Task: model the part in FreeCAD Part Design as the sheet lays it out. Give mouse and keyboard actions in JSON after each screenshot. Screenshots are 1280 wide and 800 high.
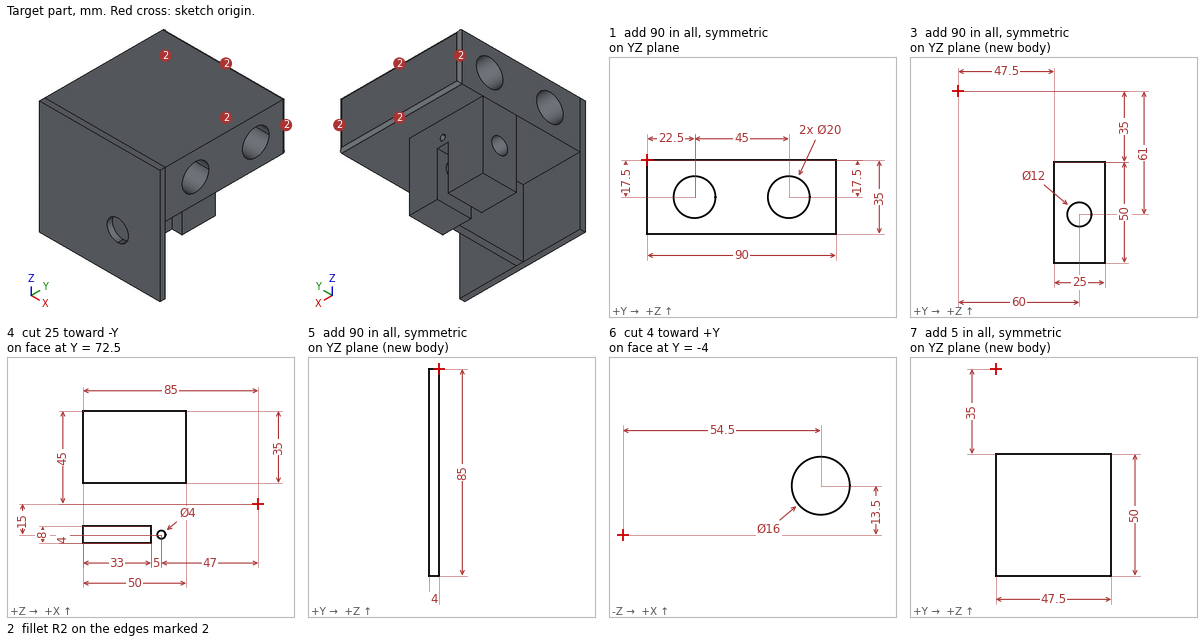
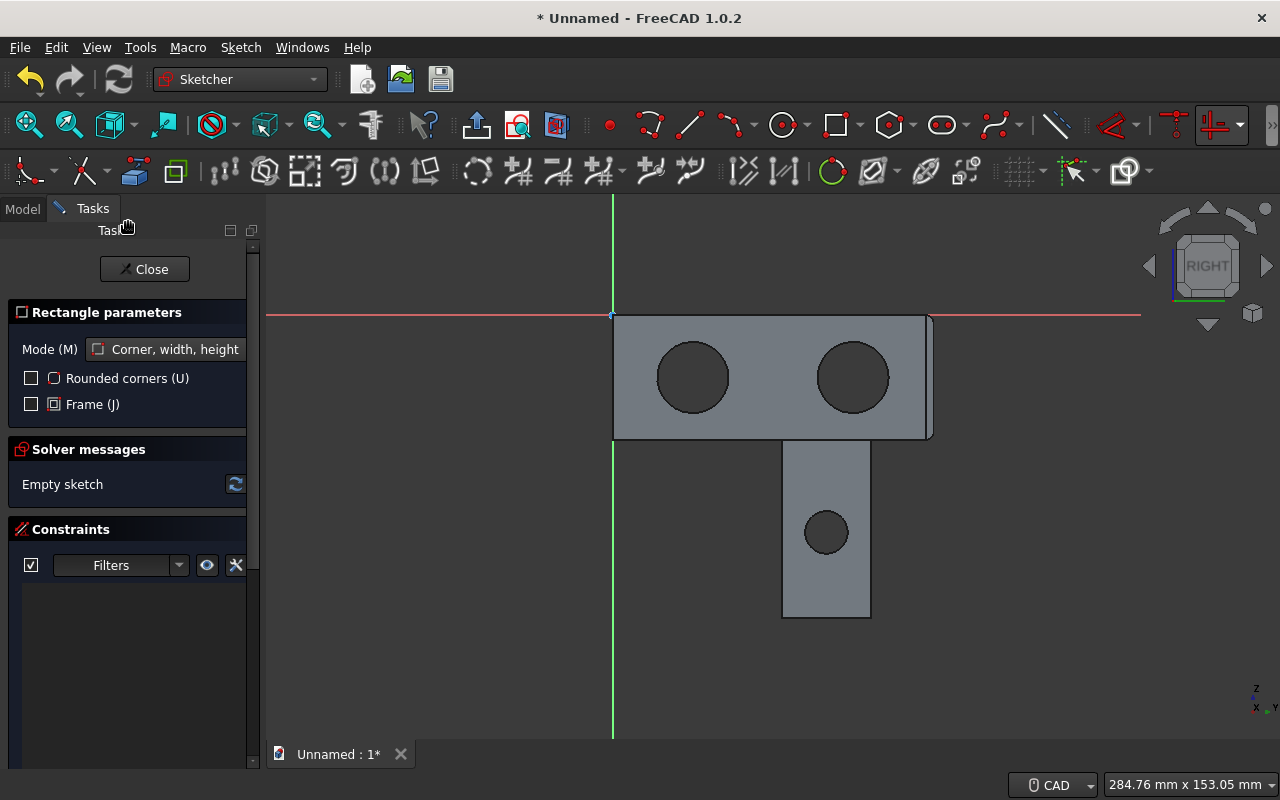
{"action": "left_click", "coordinate": [613, 315]}
{"action": "mouse_move", "coordinate": [599, 618]}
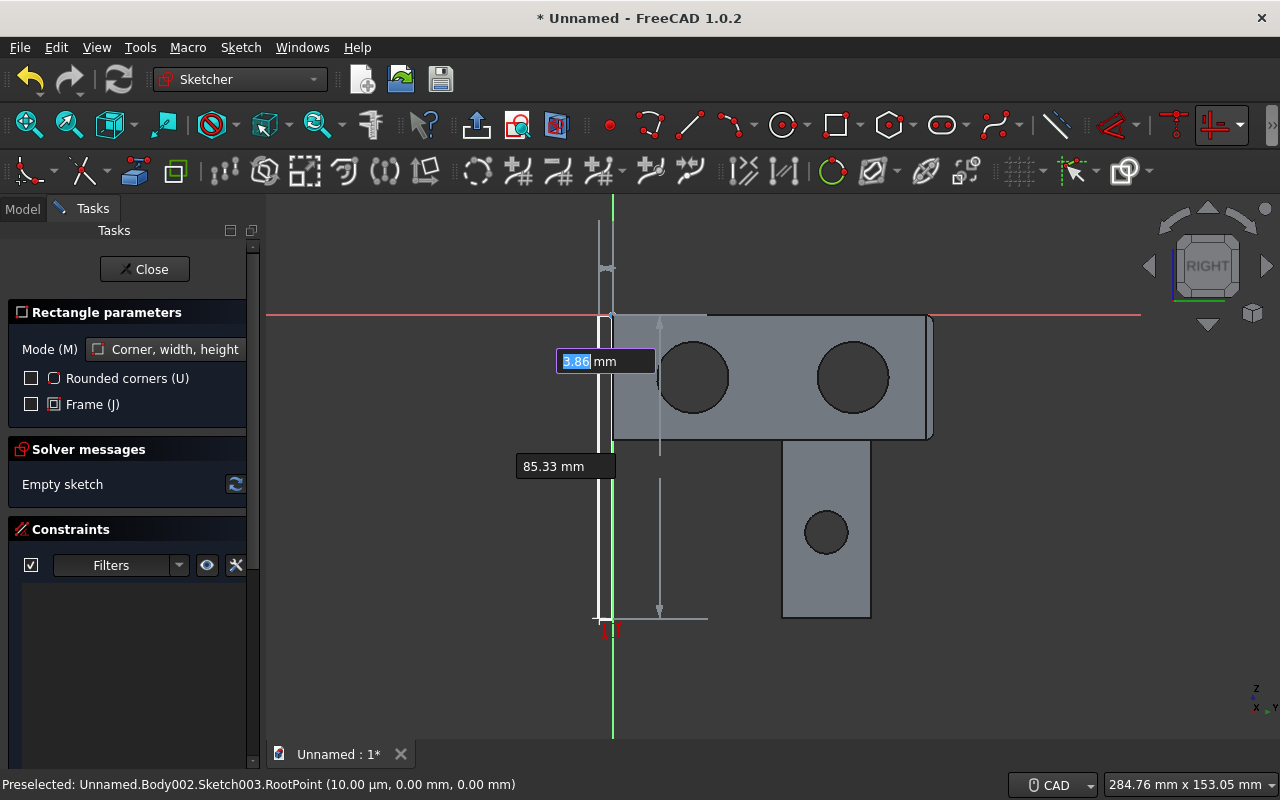
{"action": "type", "text": "4"}
{"action": "key", "text": "Tab"}
{"action": "type", "text": "85"}
{"action": "key", "text": "Return"}
{"action": "key", "text": "Escape"}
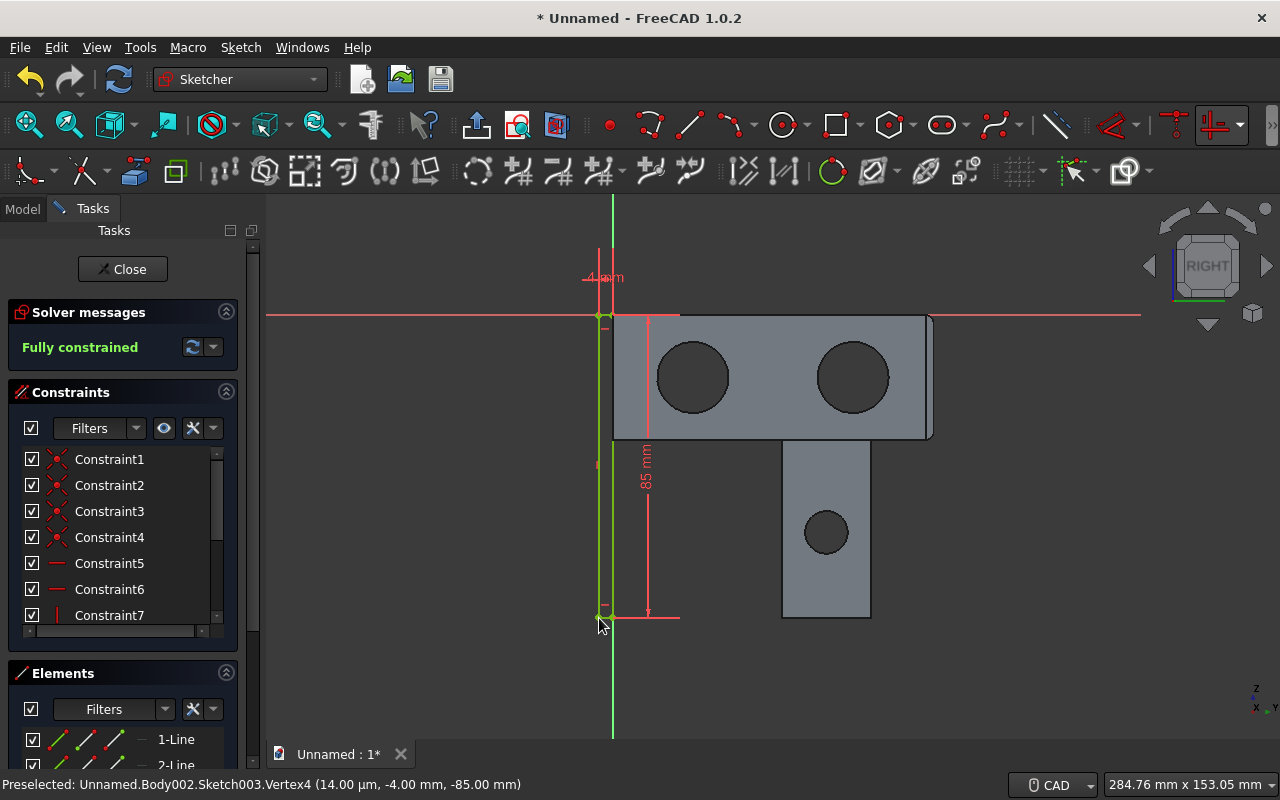
{"action": "left_click", "coordinate": [123, 269]}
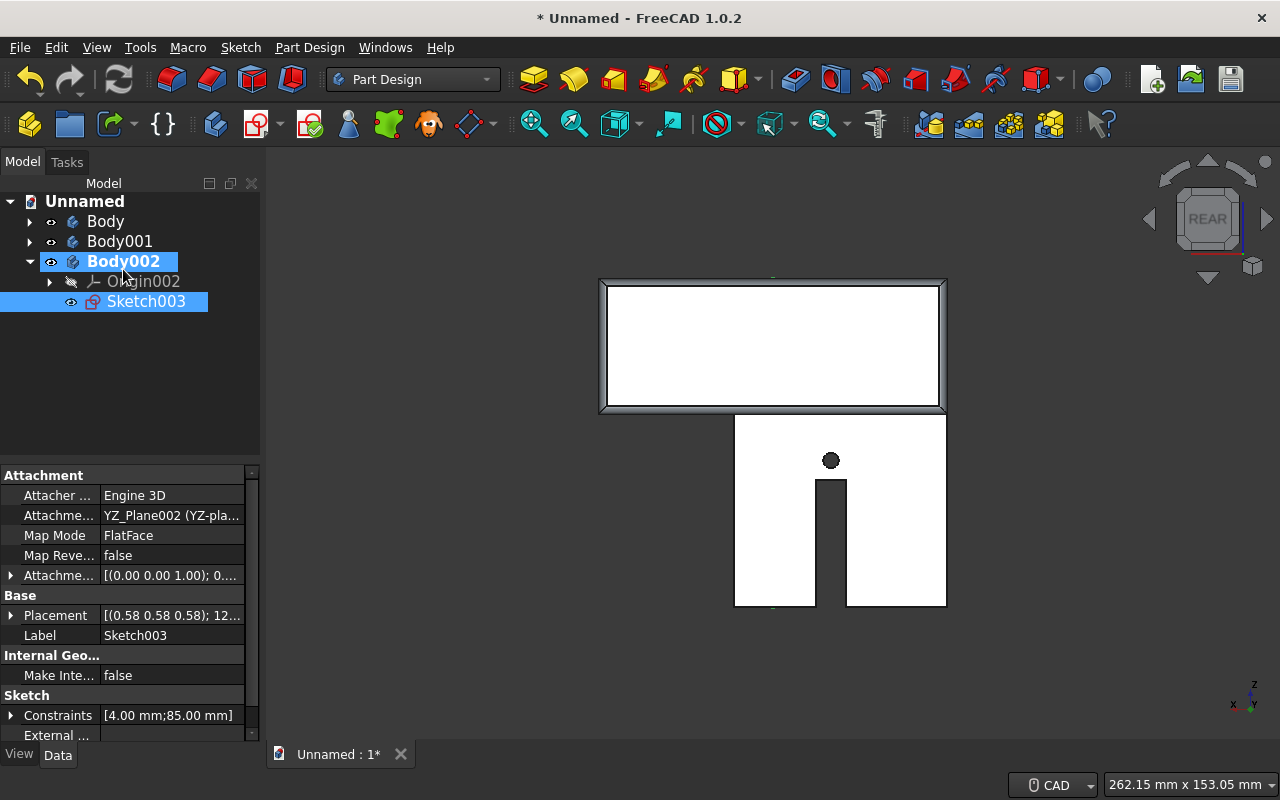
{"action": "left_click", "coordinate": [534, 80]}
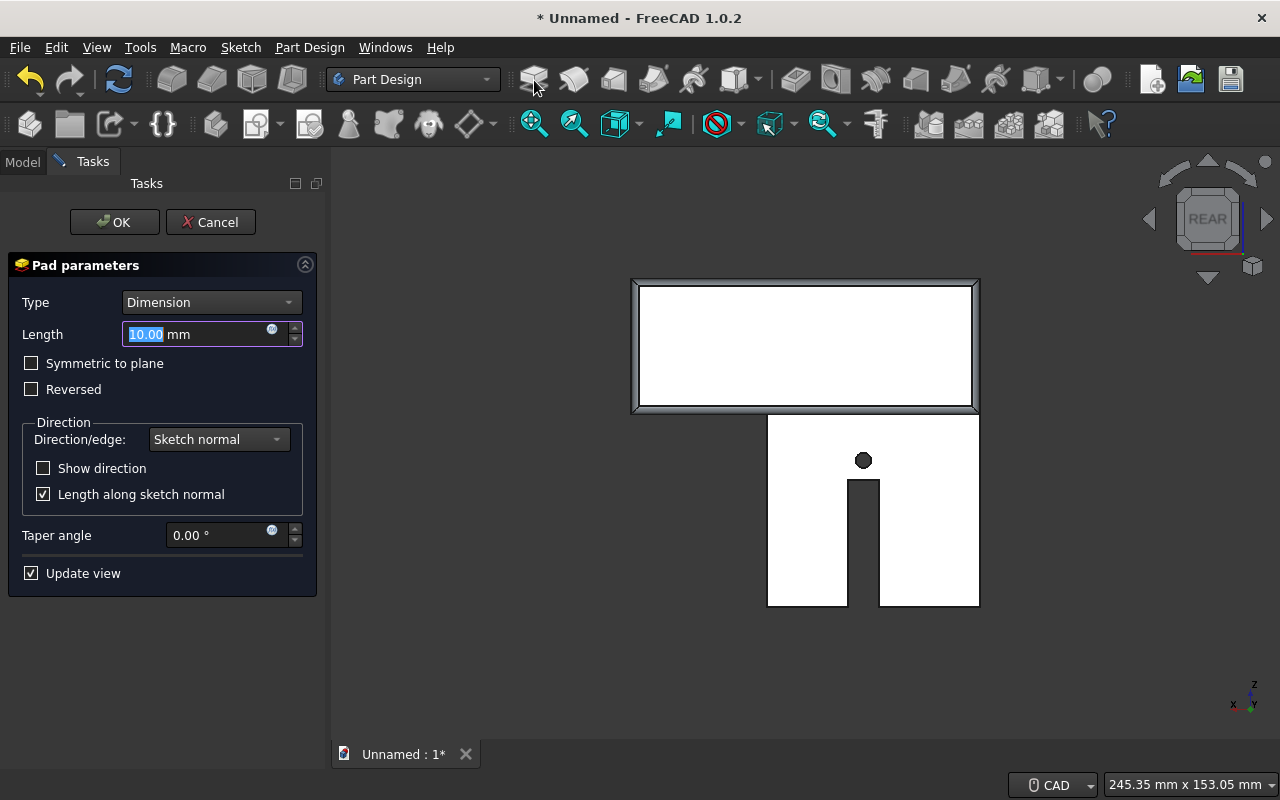
{"action": "type", "text": "90"}
{"action": "key", "text": "Tab"}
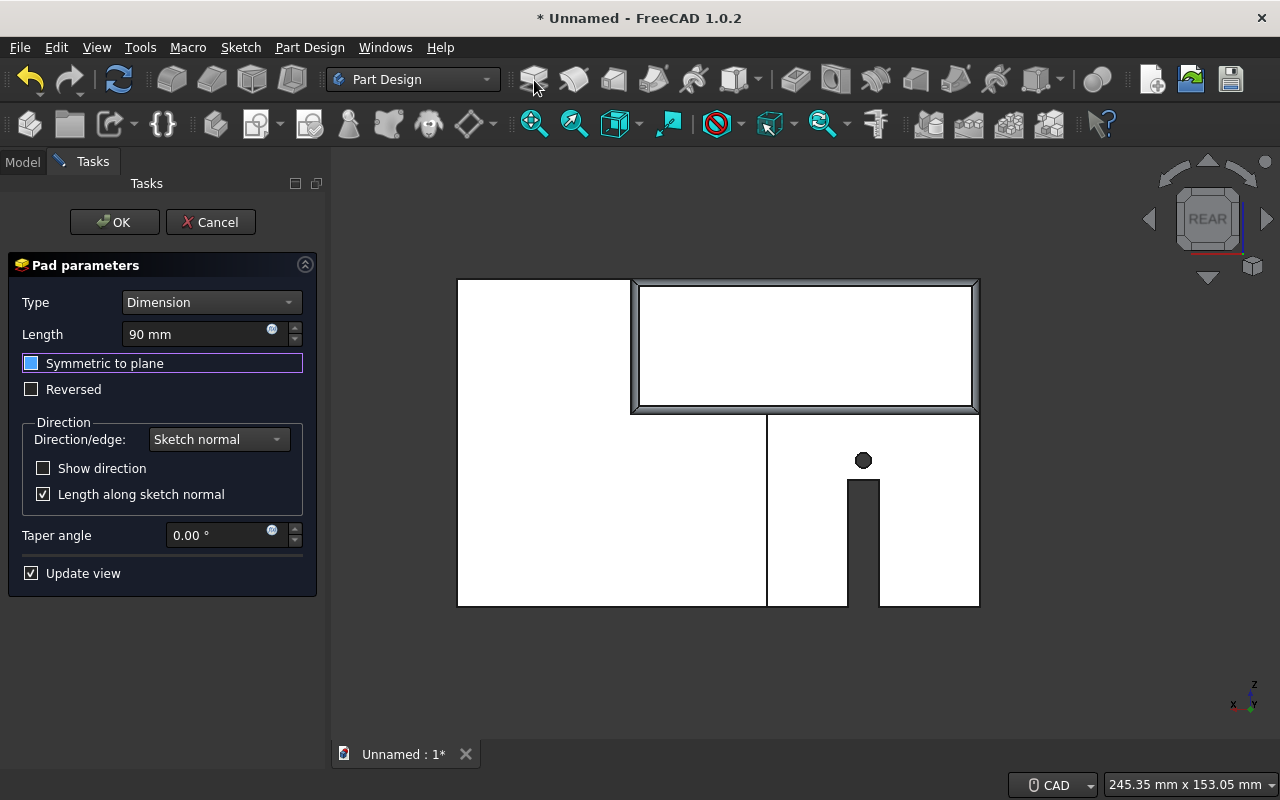
{"action": "left_click", "coordinate": [30, 363]}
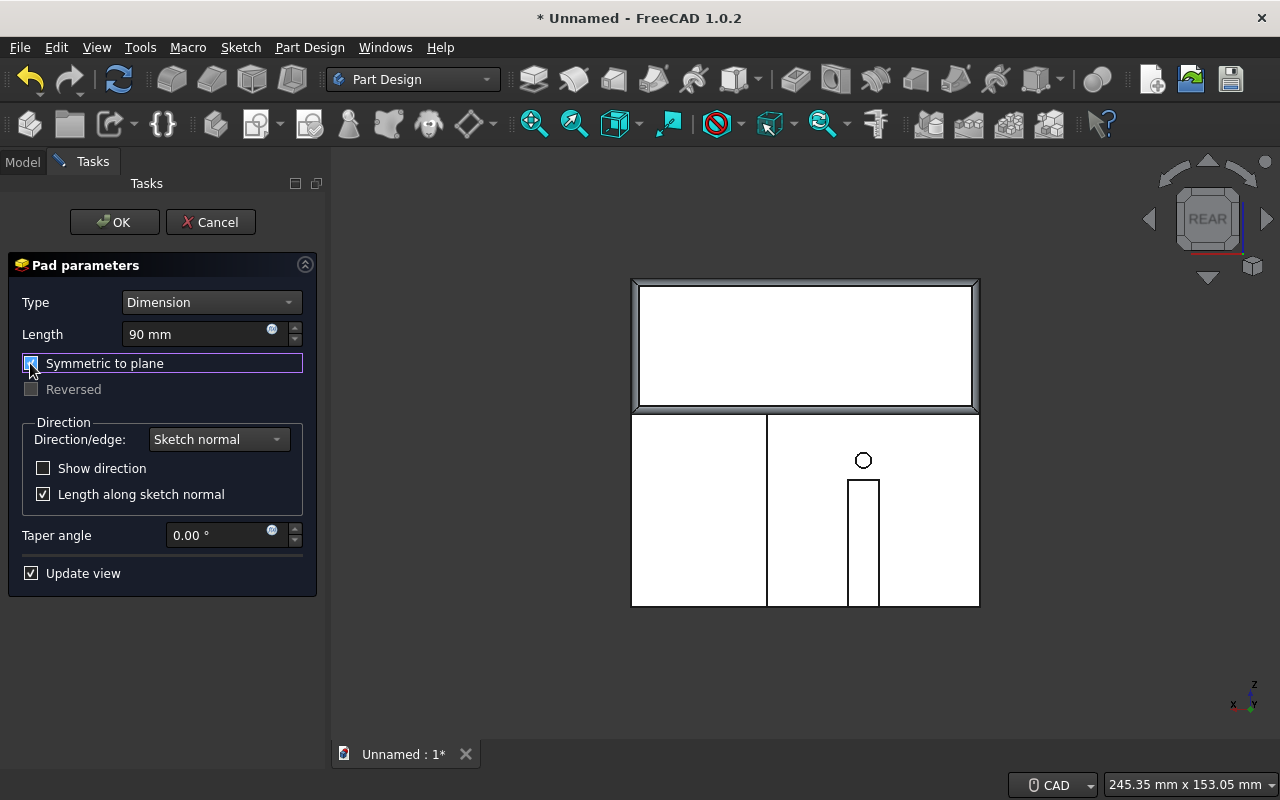
{"action": "left_click", "coordinate": [115, 222]}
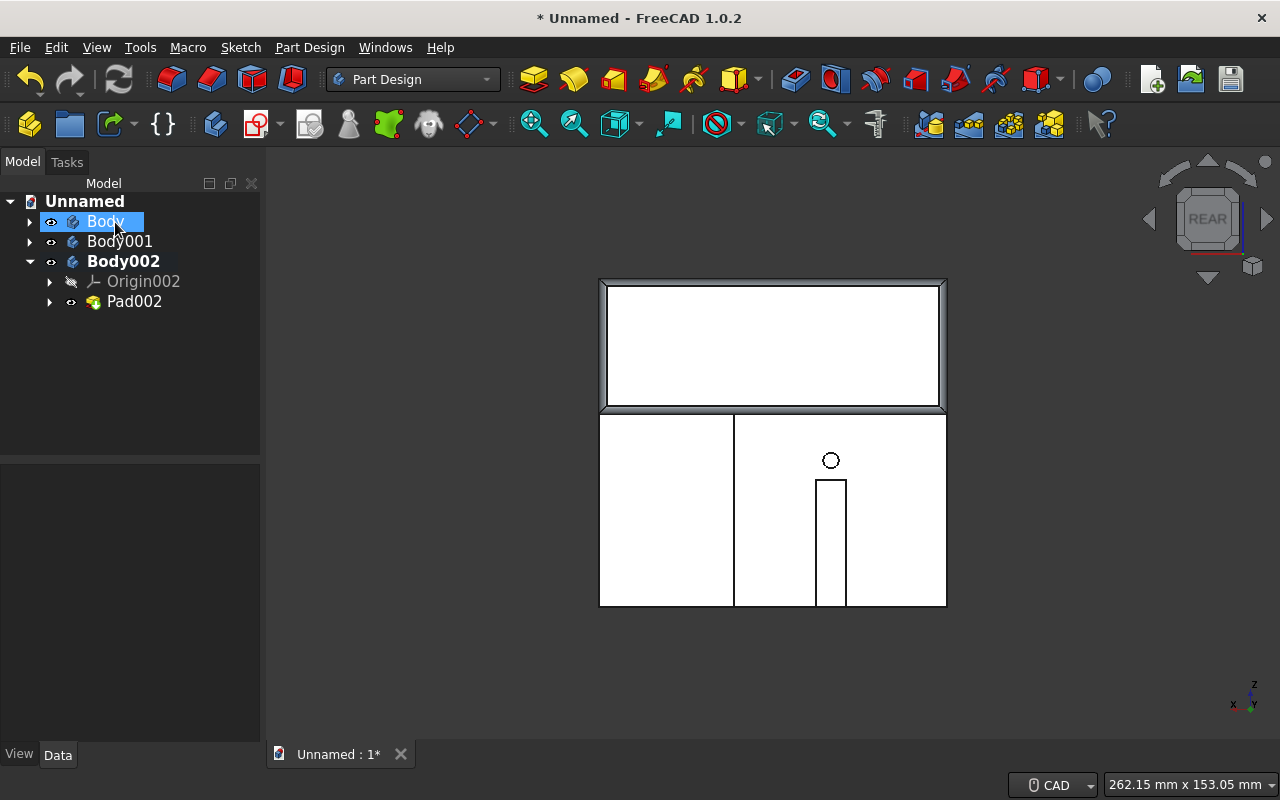
{"action": "key", "text": "0"}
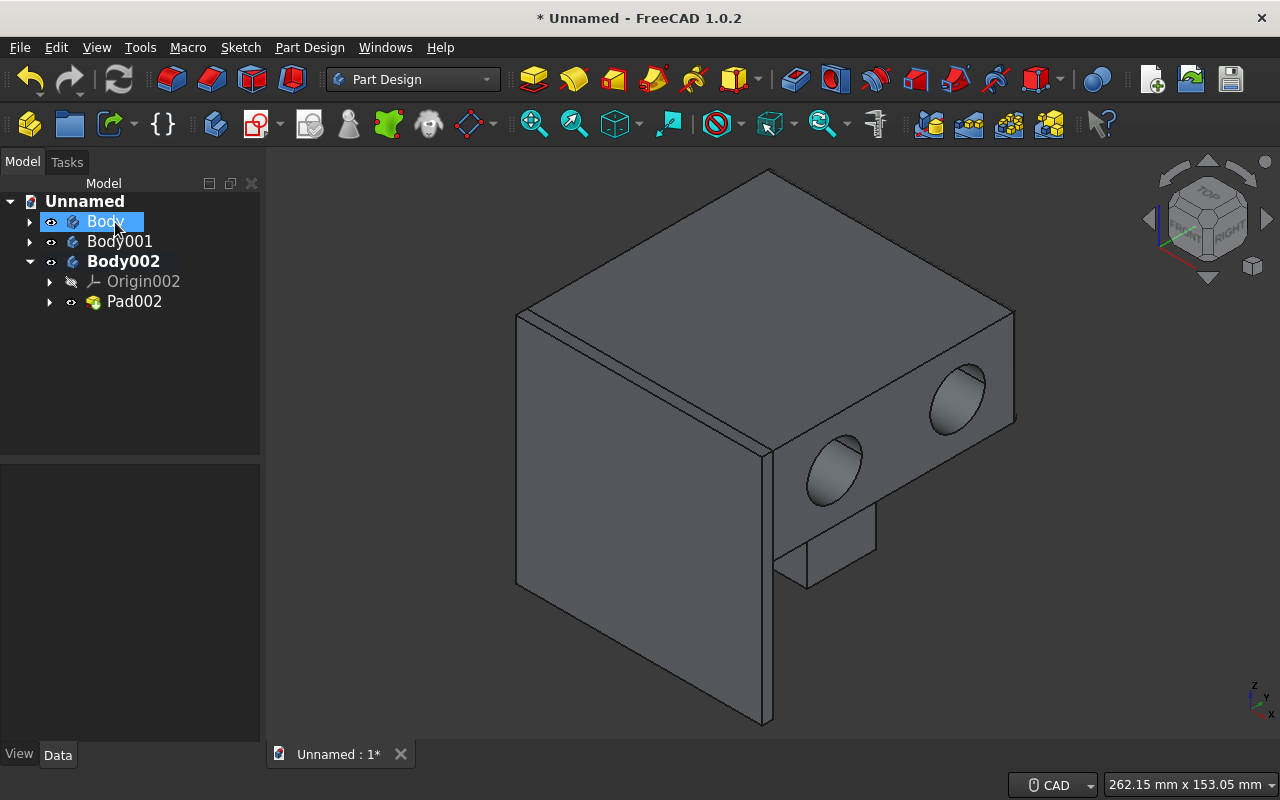
{"action": "left_click", "coordinate": [639, 519]}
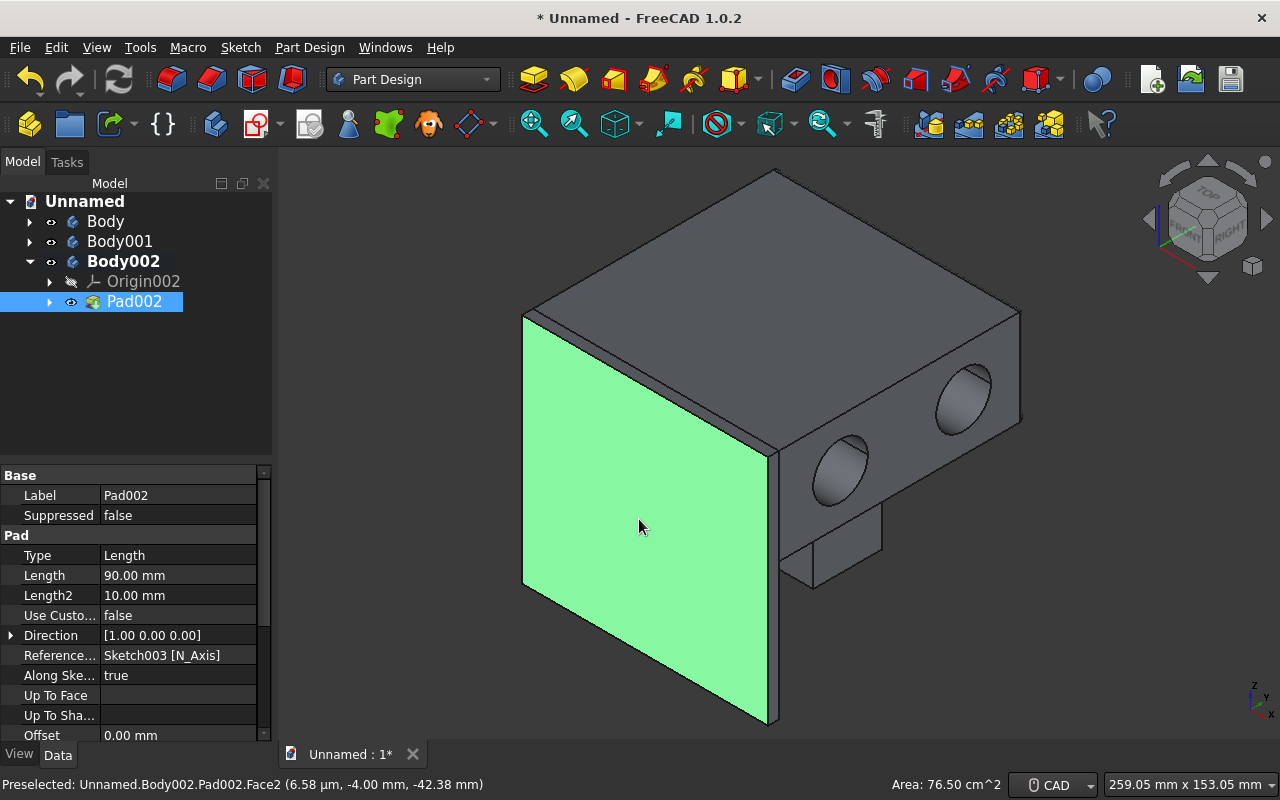
{"action": "left_click", "coordinate": [256, 124]}